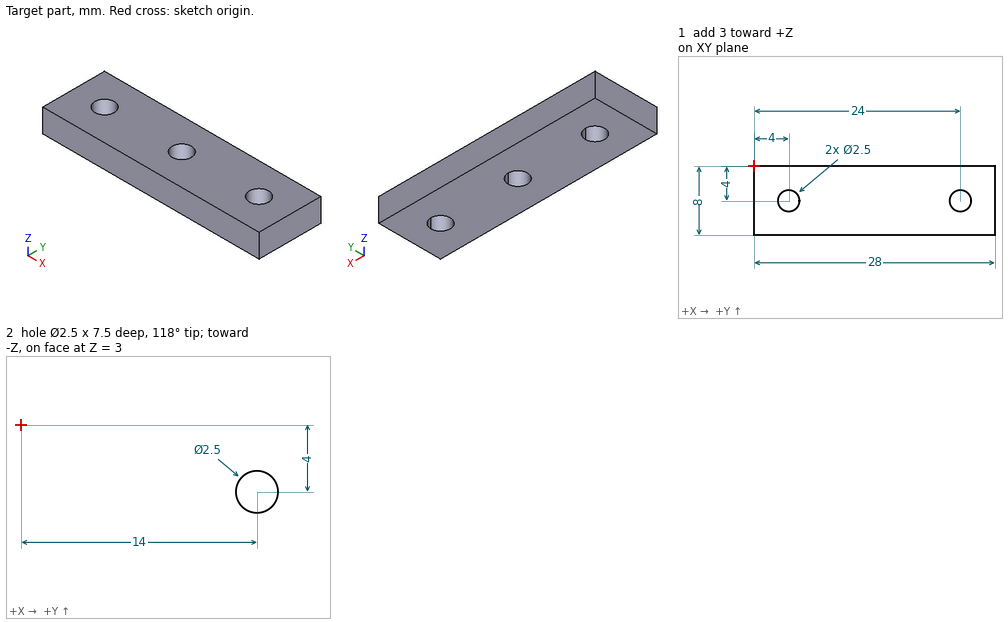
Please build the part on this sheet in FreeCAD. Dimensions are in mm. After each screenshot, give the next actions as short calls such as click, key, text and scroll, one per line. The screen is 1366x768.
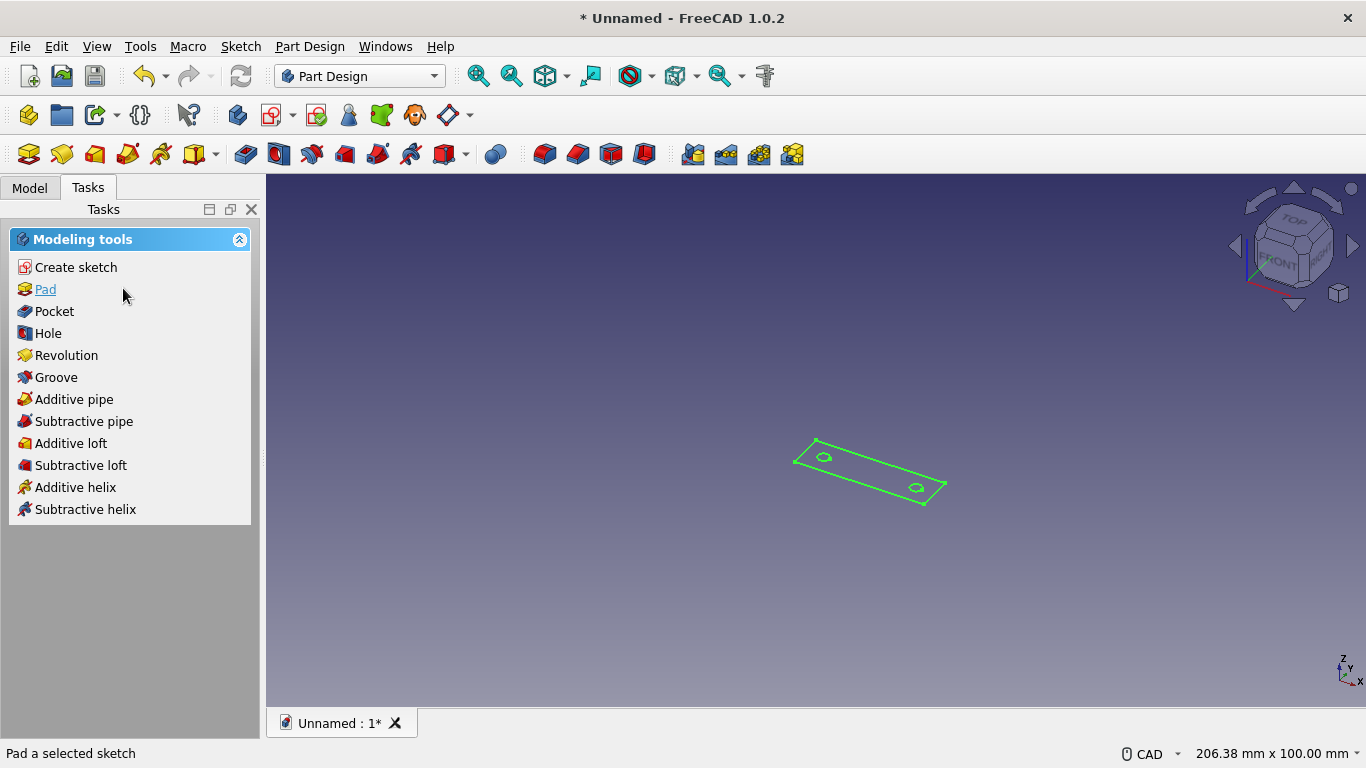
click(29, 154)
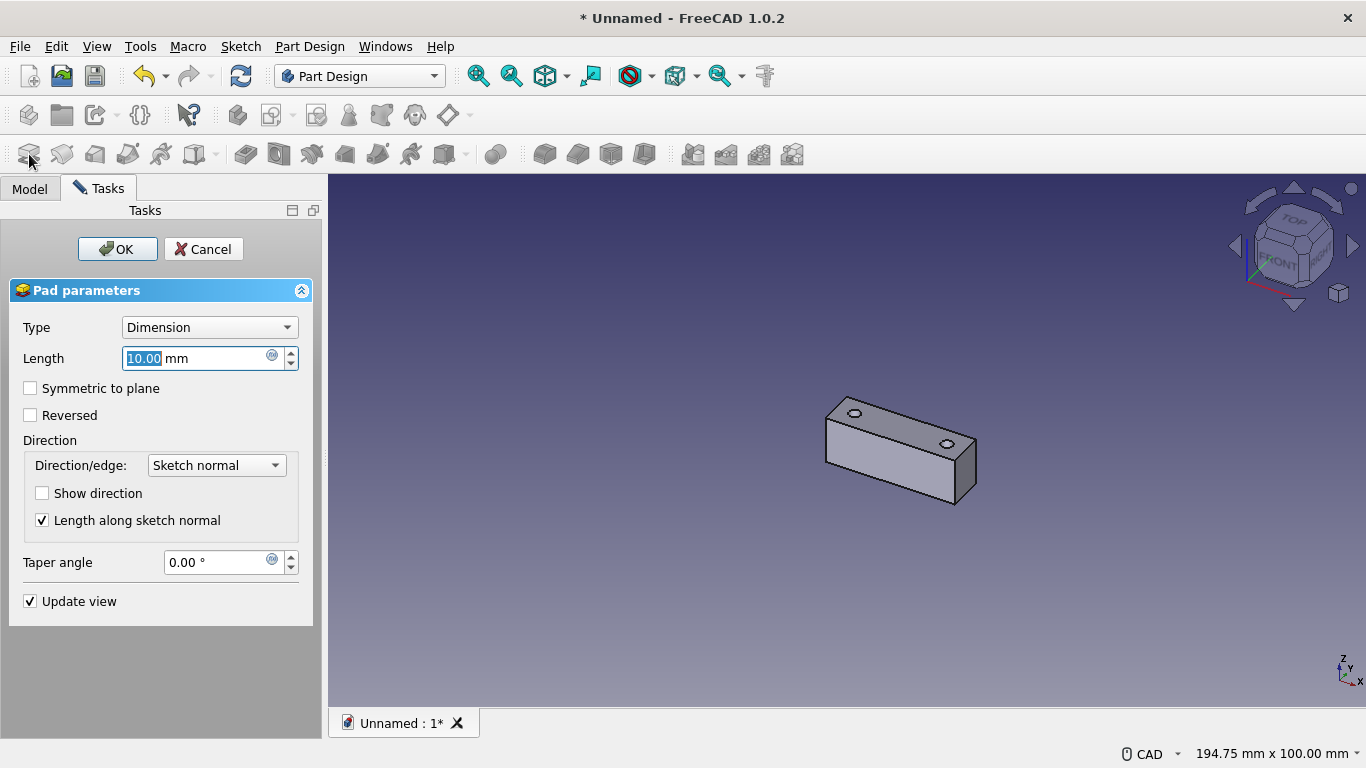
text(3)
key(Tab)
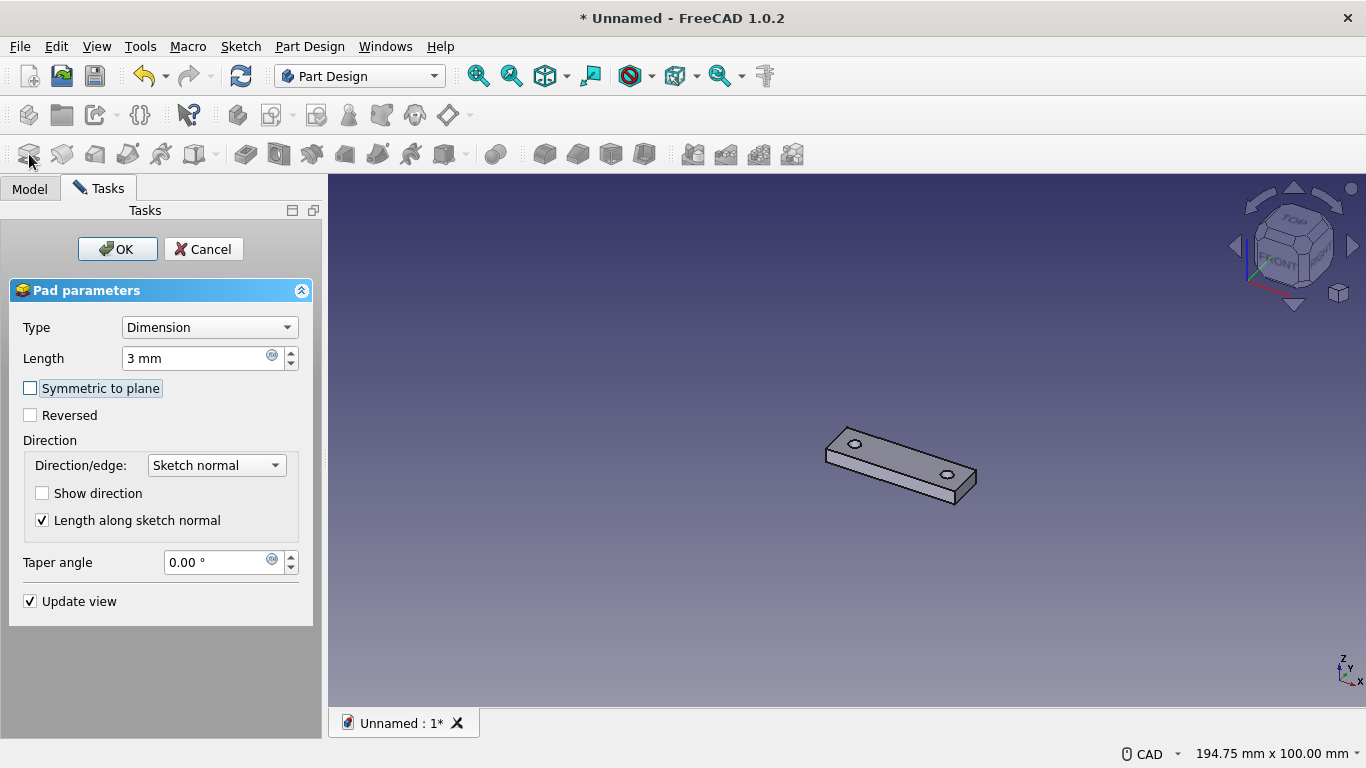
click(118, 249)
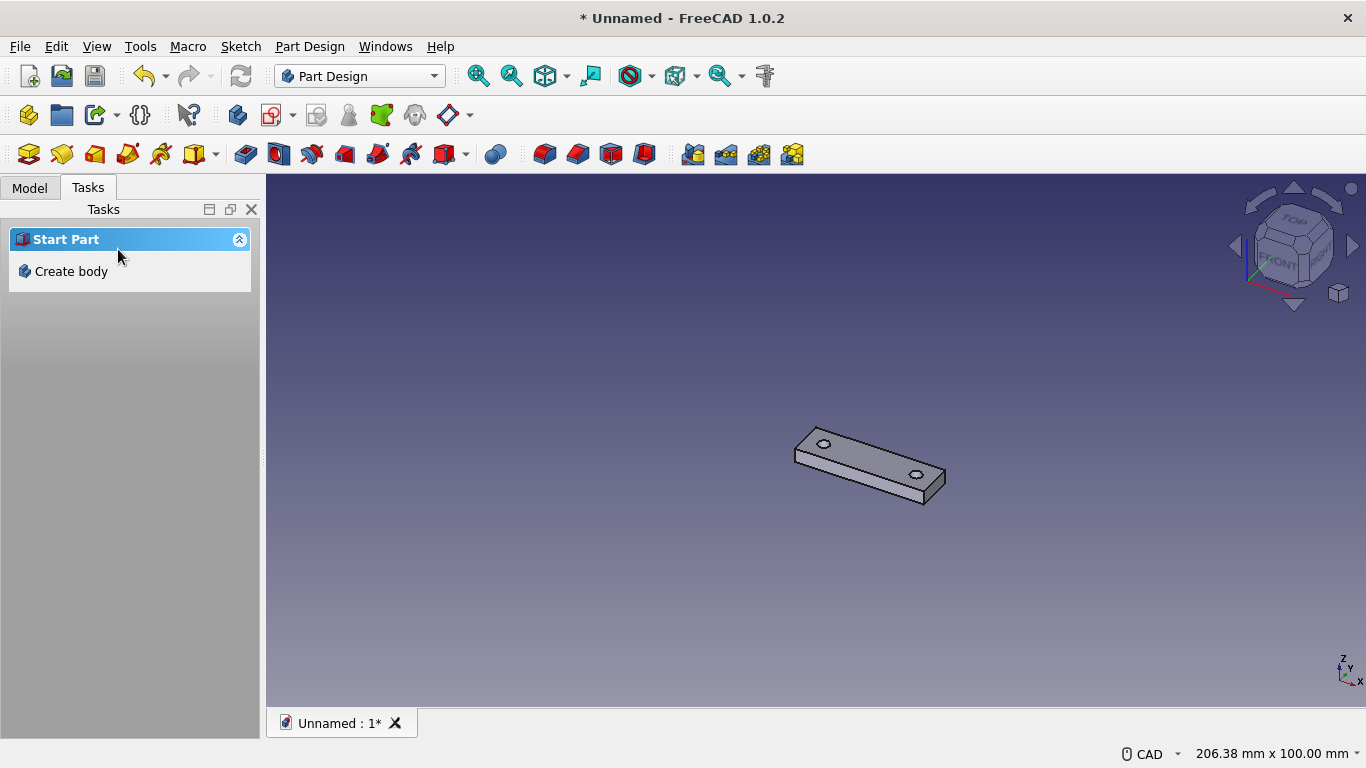
click(479, 76)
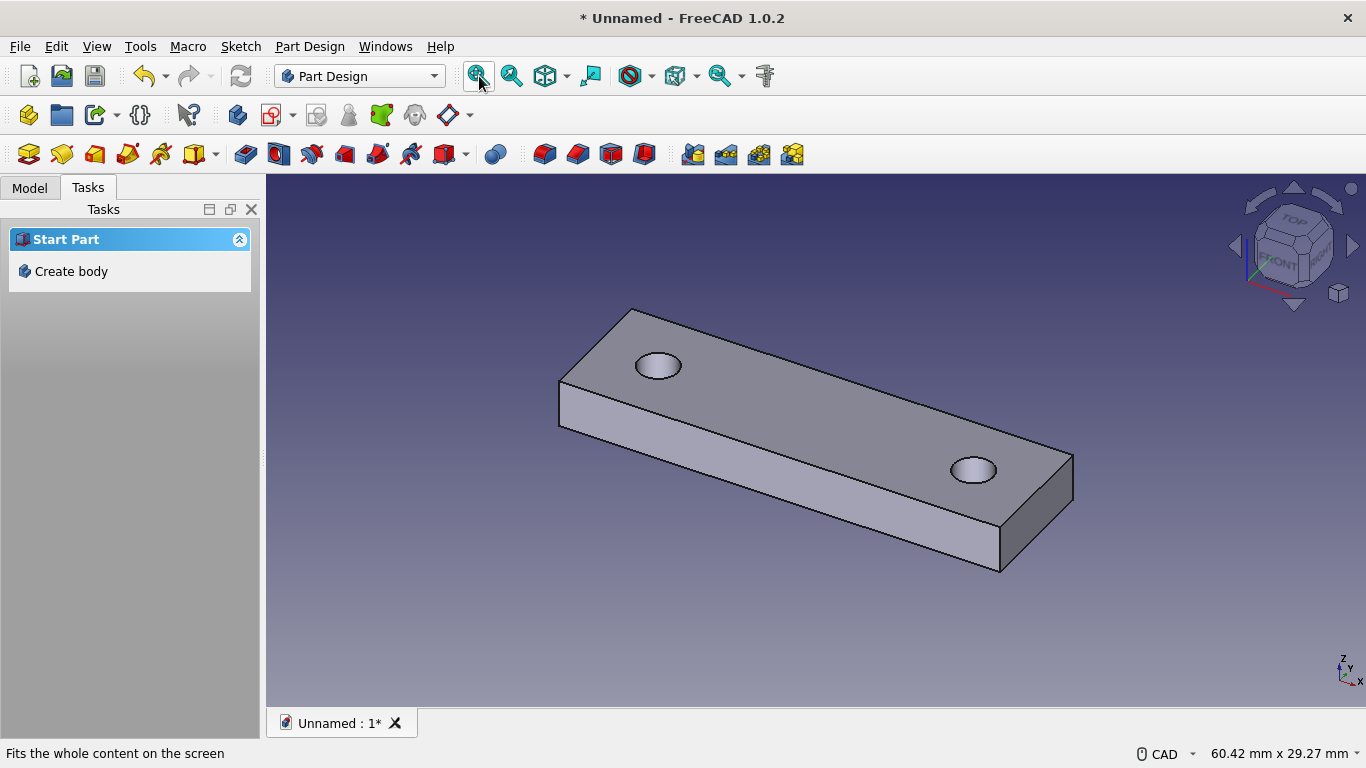
click(879, 438)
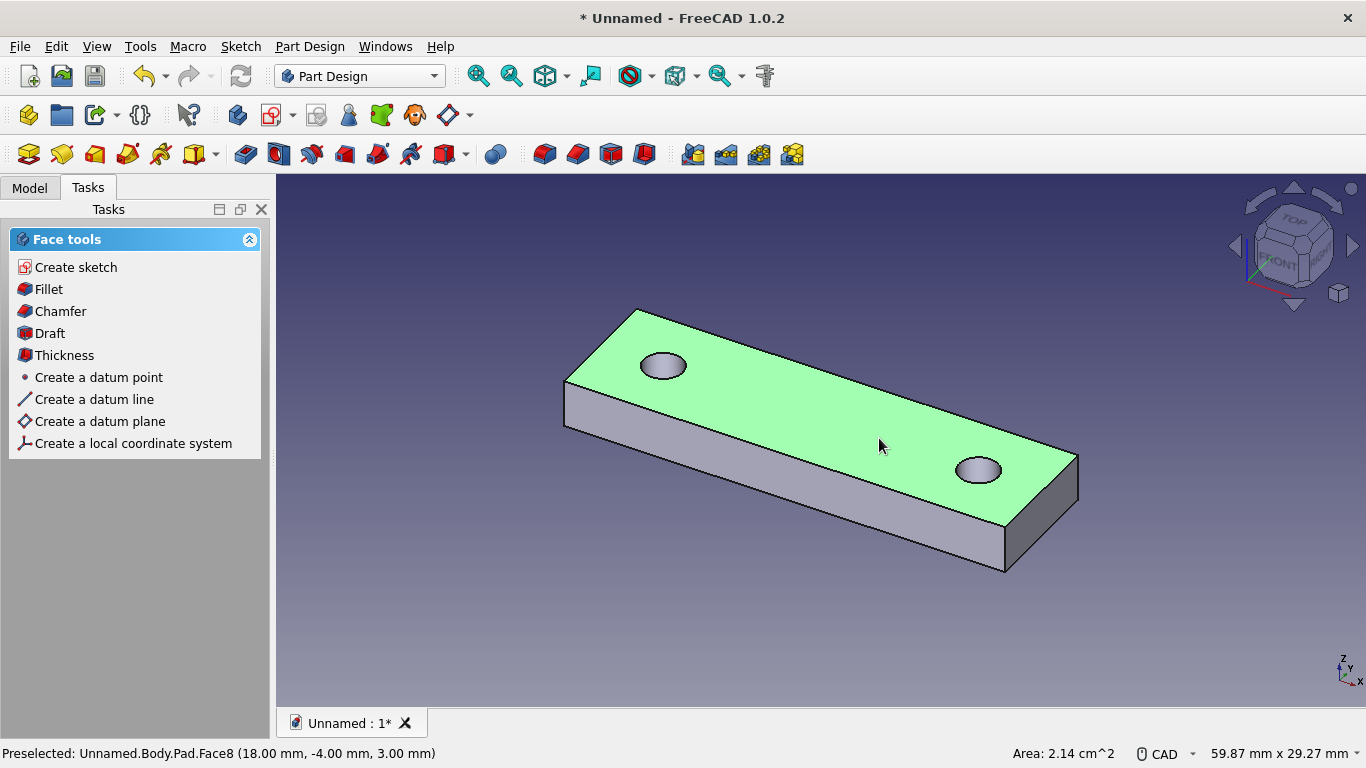
click(270, 116)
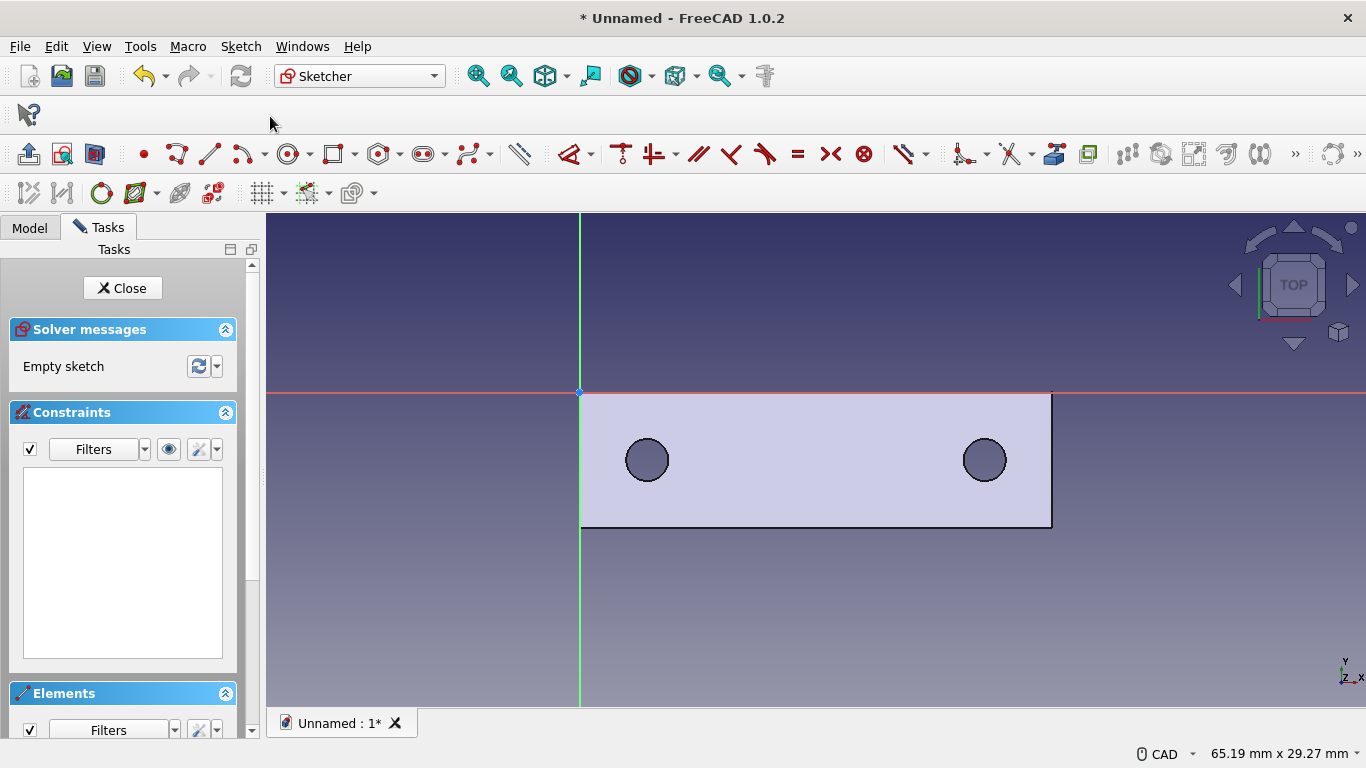
scroll(827, 460, up, 10)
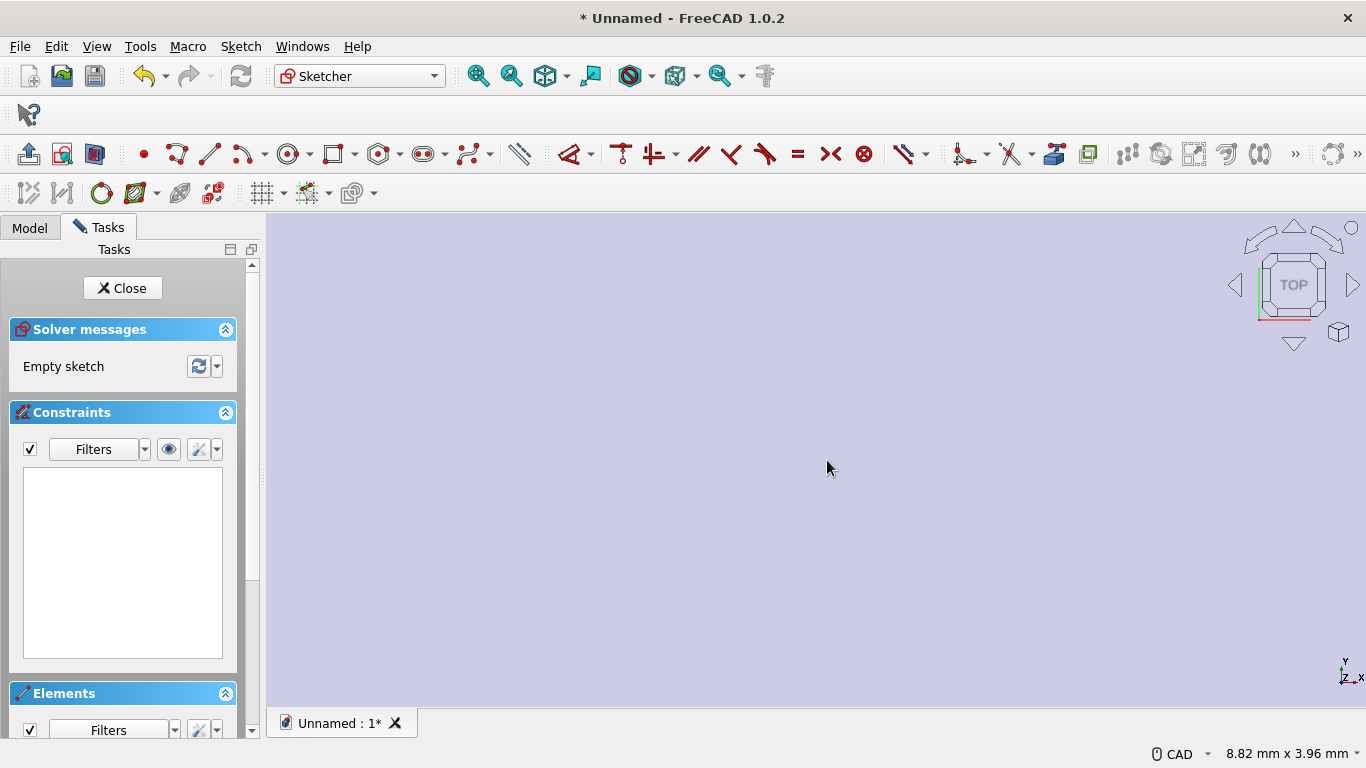
click(288, 154)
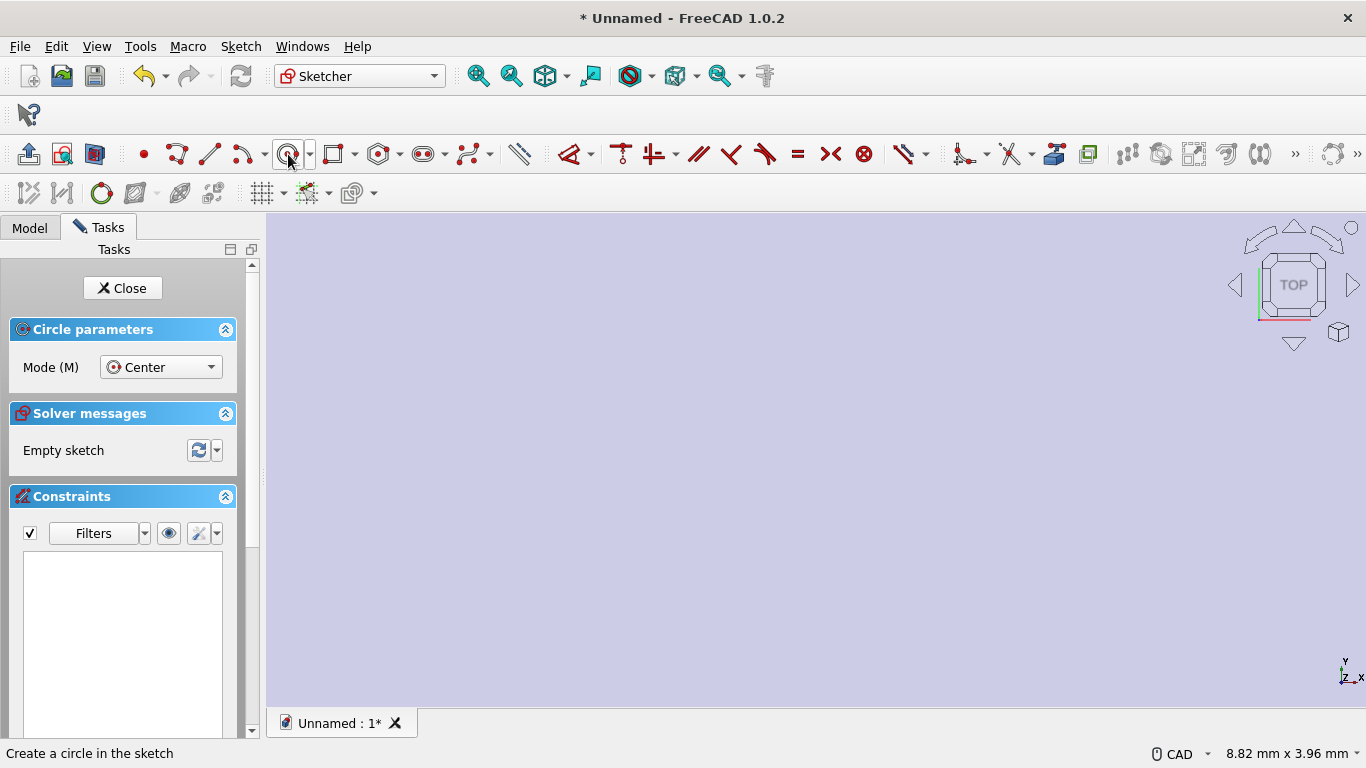
click(742, 457)
click(853, 347)
key(Escape)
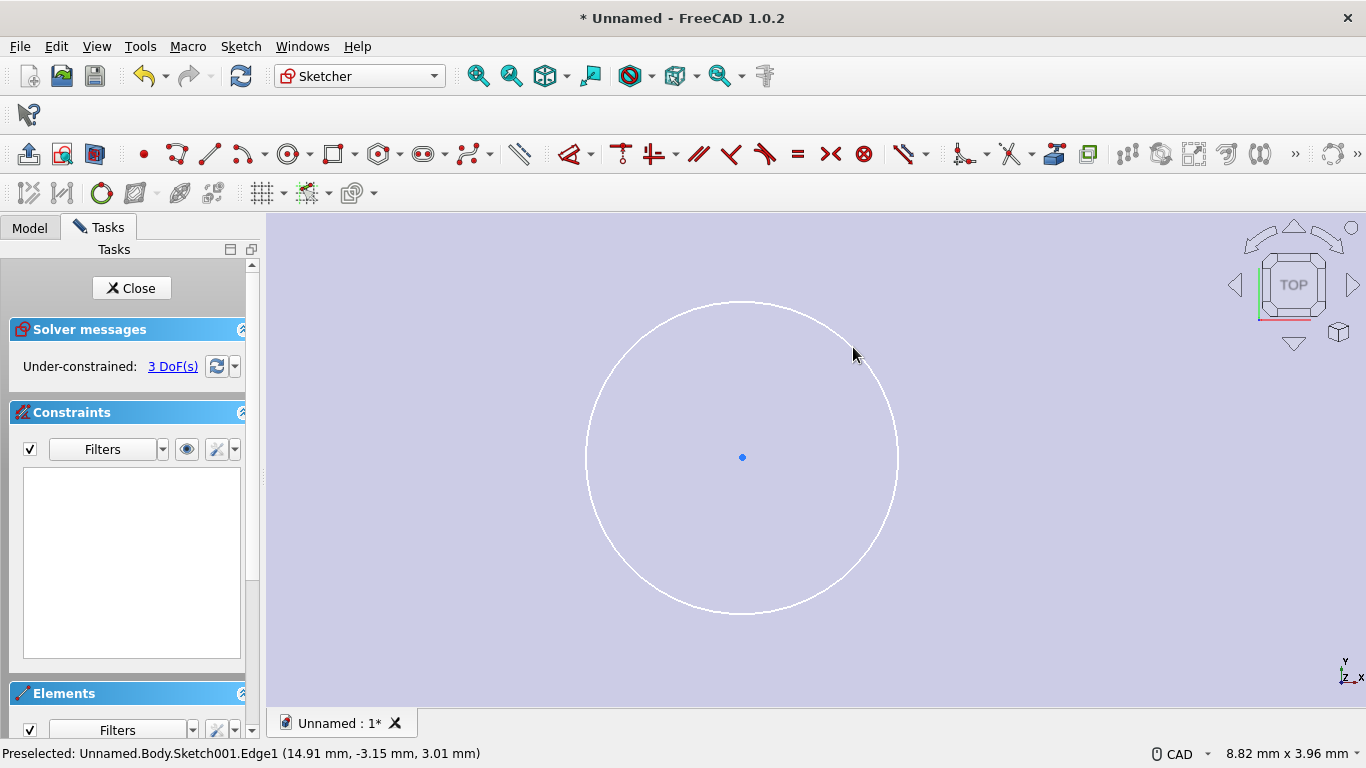
key(d)